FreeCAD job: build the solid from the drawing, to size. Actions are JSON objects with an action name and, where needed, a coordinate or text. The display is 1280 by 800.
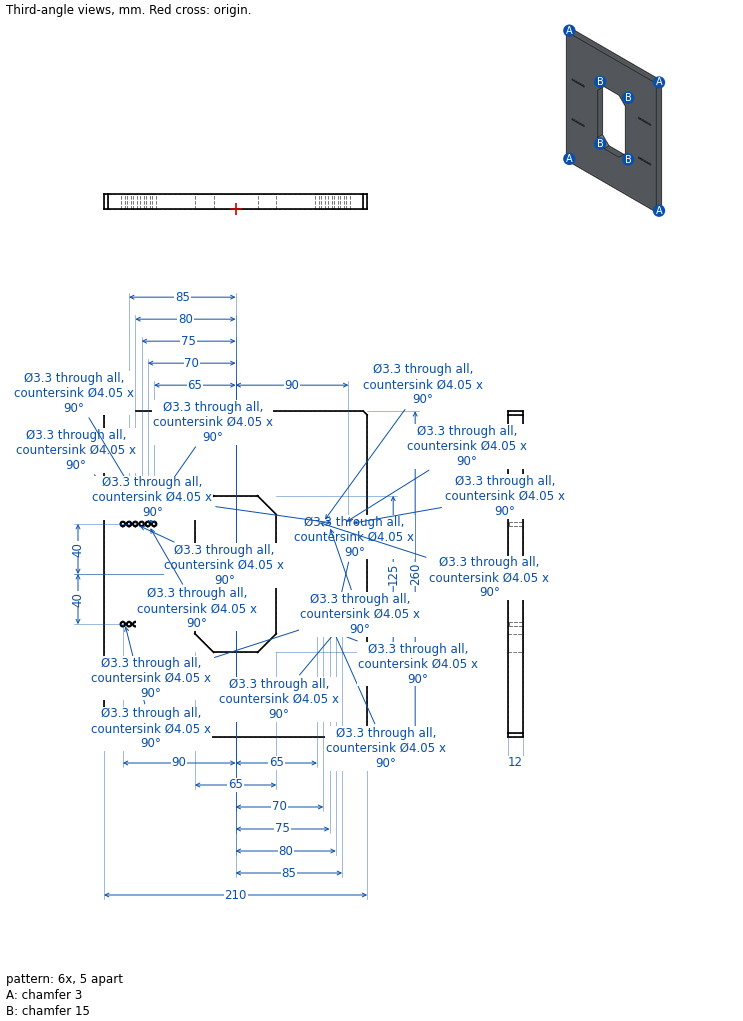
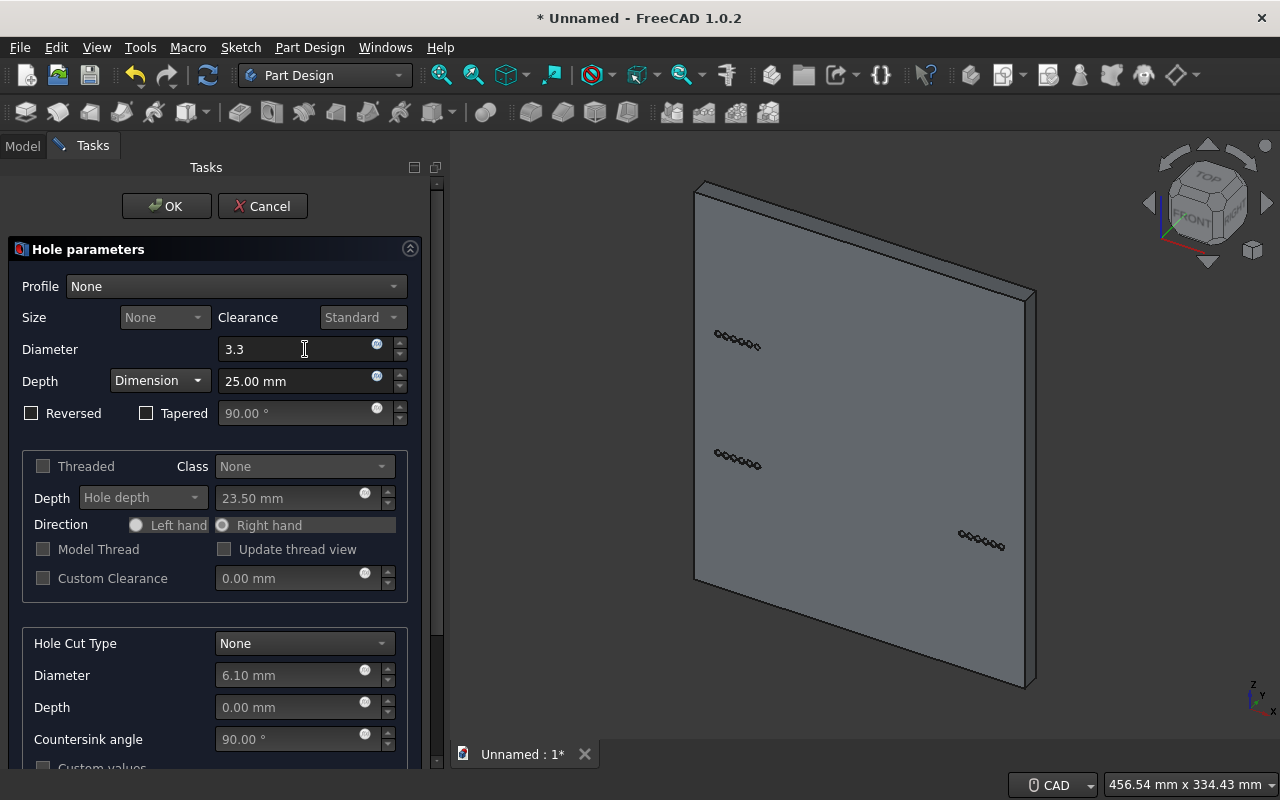
{"action": "left_click", "coordinate": [161, 380]}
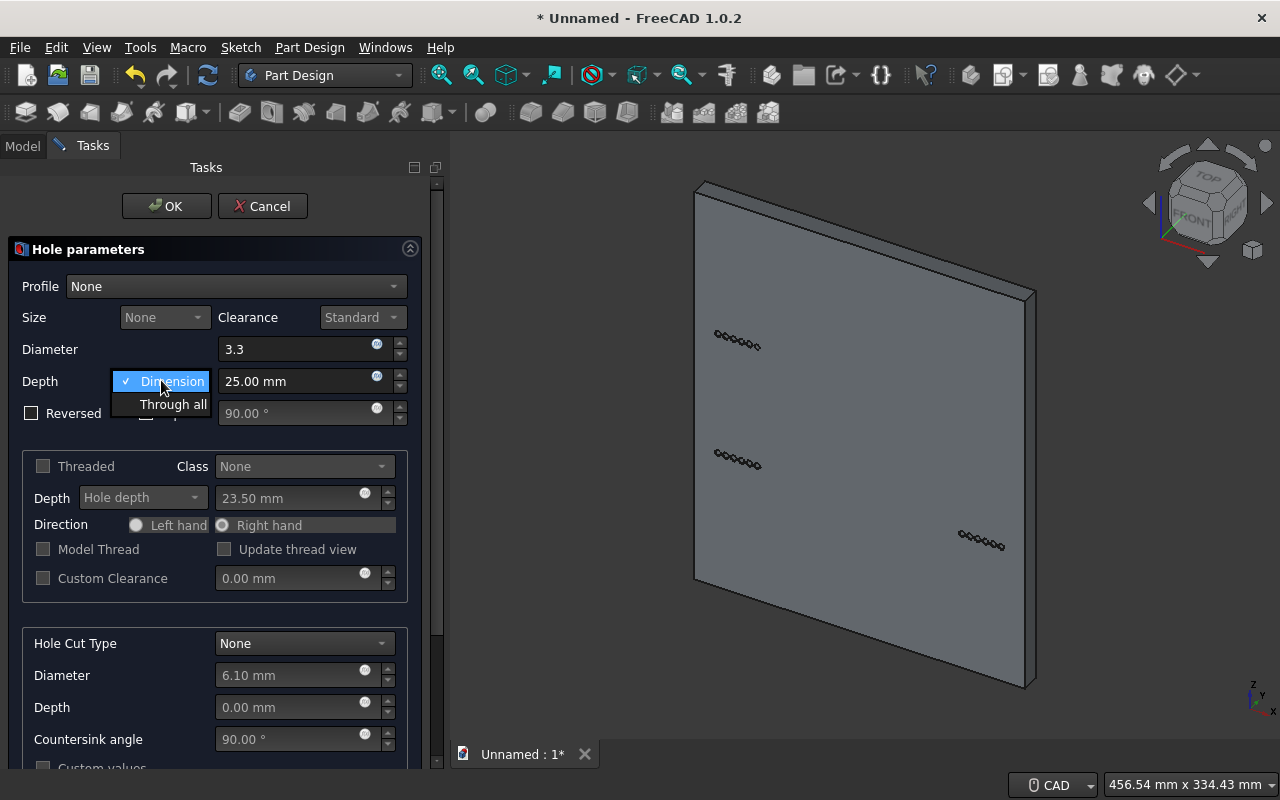
{"action": "left_click", "coordinate": [160, 404]}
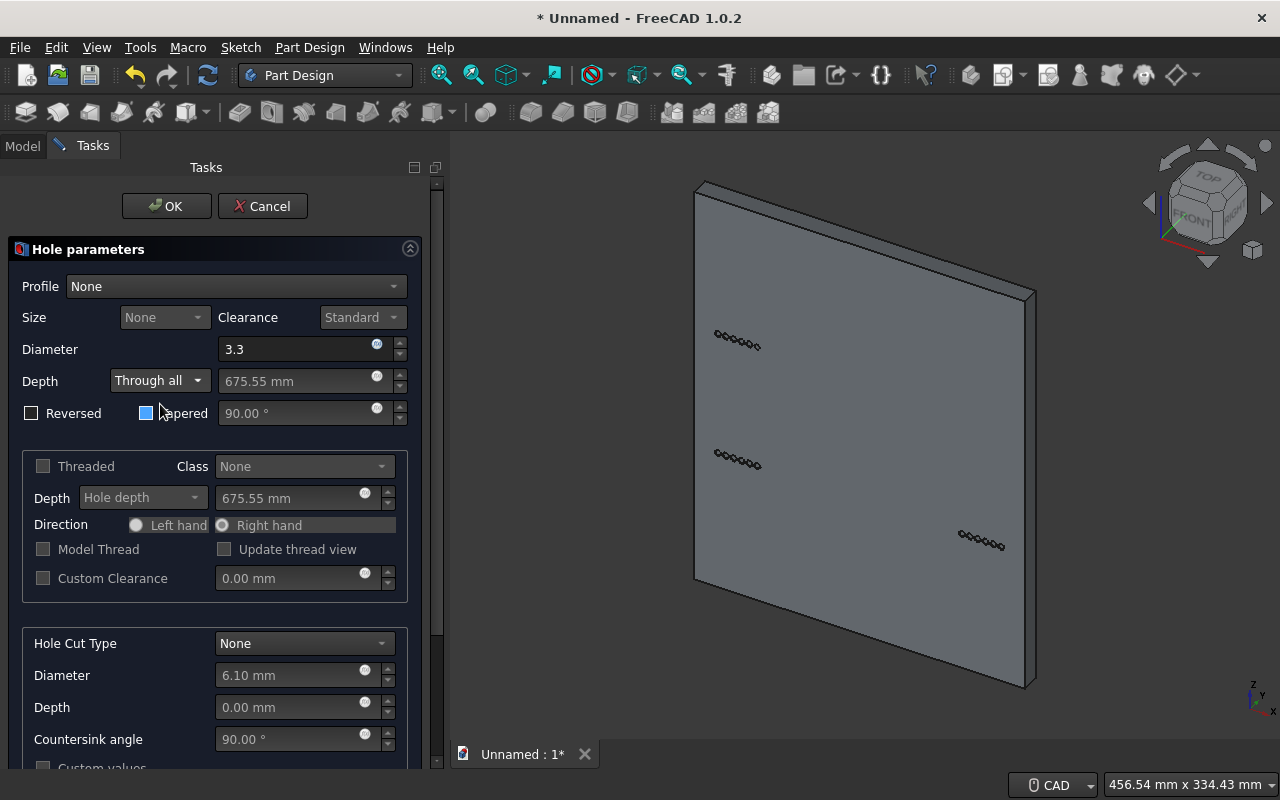
{"action": "left_click", "coordinate": [306, 644]}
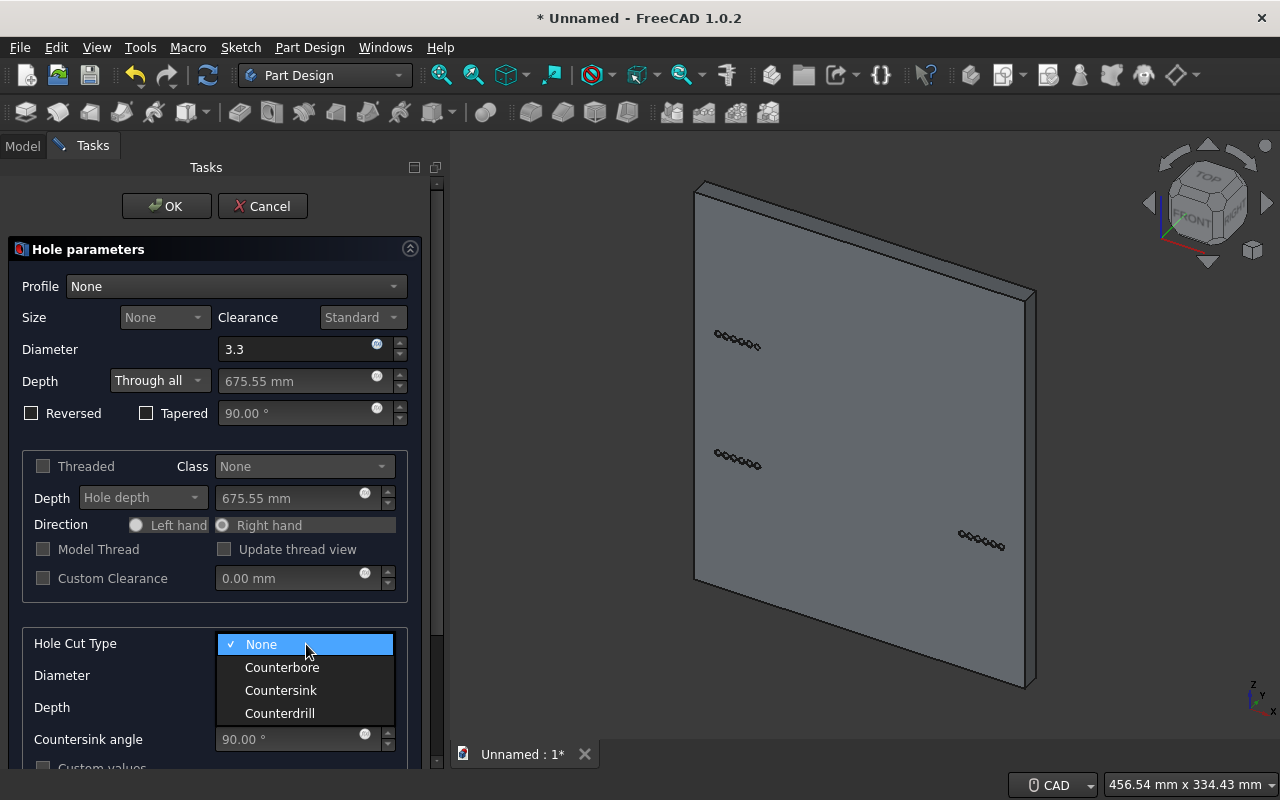
{"action": "left_click", "coordinate": [304, 690]}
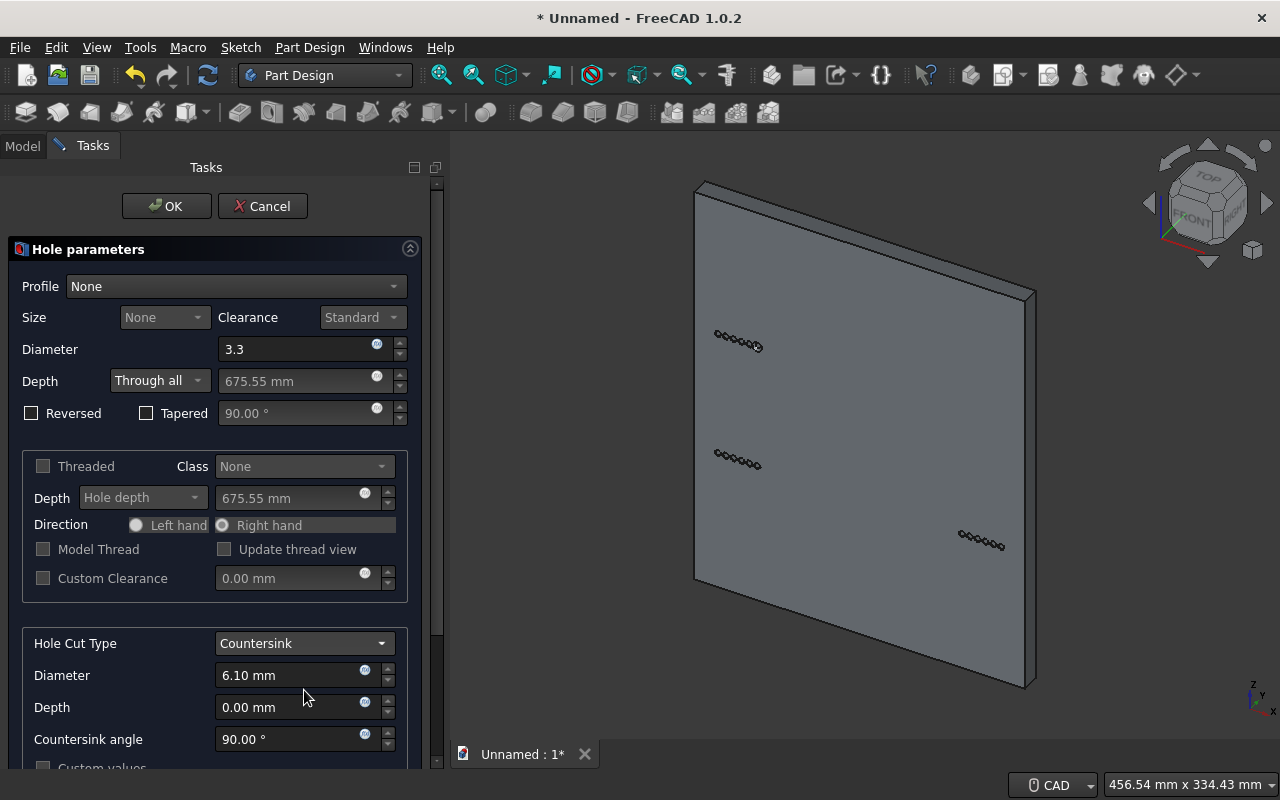
{"action": "triple_click", "coordinate": [298, 675]}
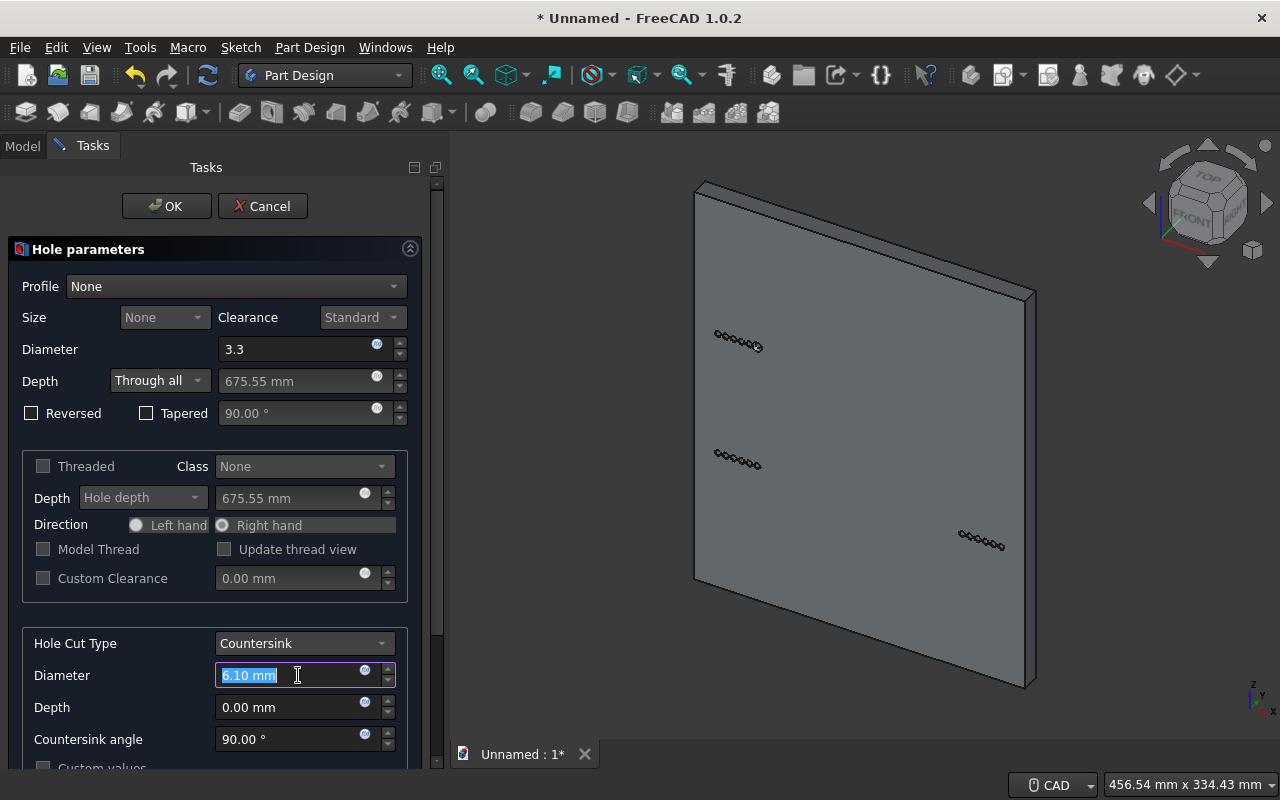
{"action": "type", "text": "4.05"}
{"action": "key", "text": "Tab"}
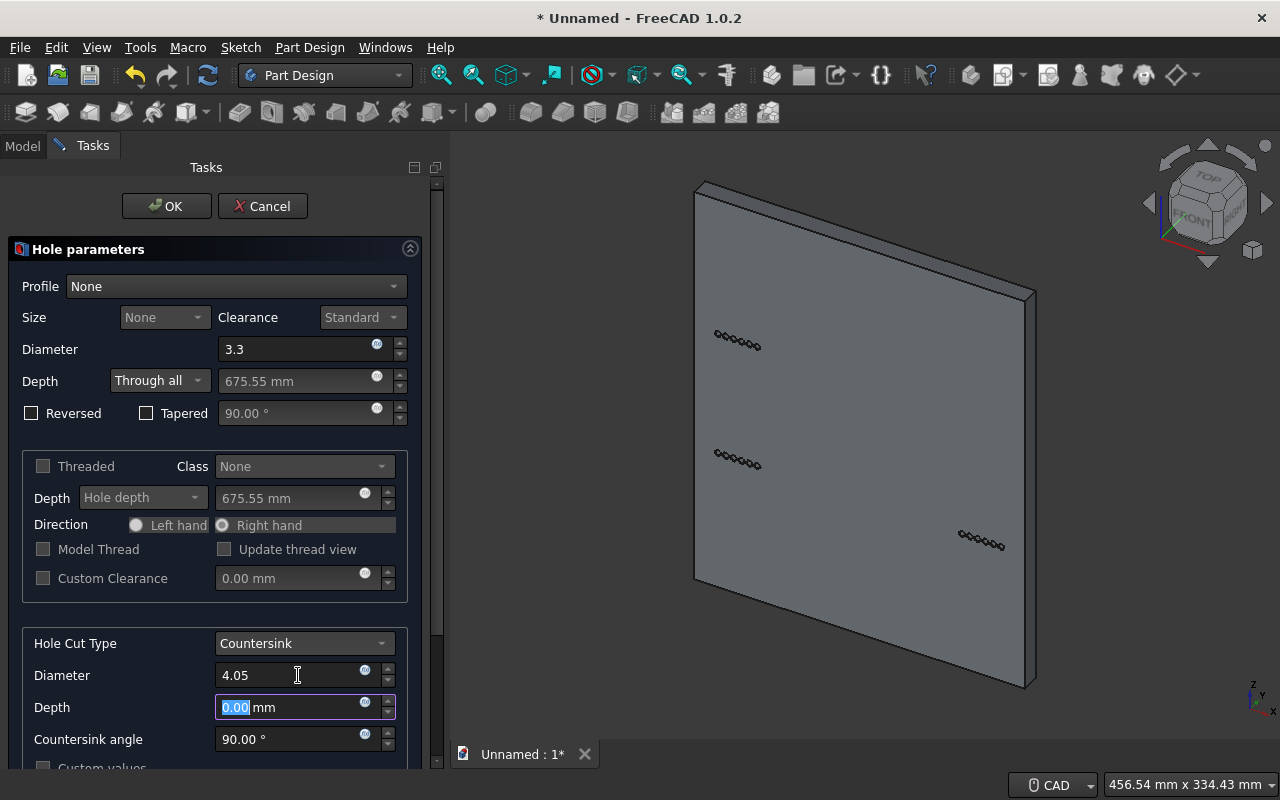
{"action": "left_click", "coordinate": [167, 206]}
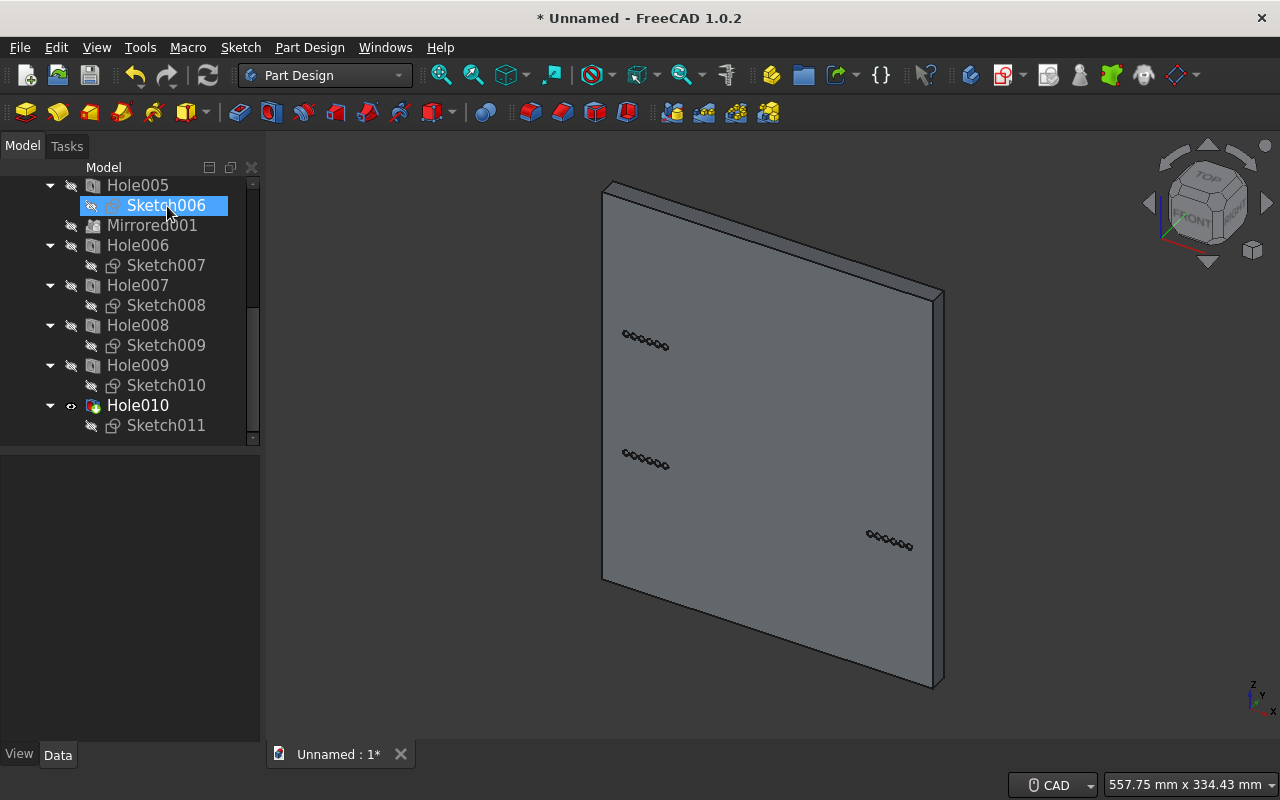
{"action": "left_click", "coordinate": [815, 400]}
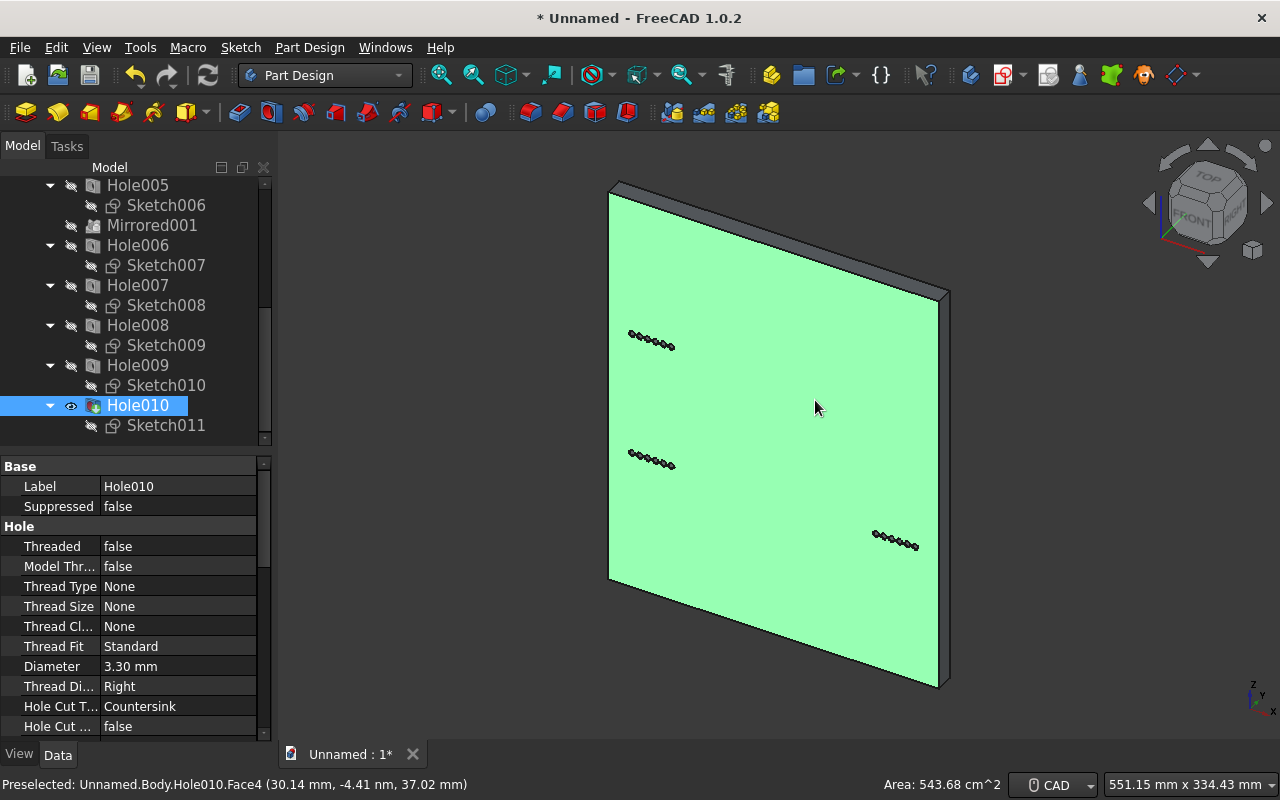
{"action": "left_click", "coordinate": [1004, 76]}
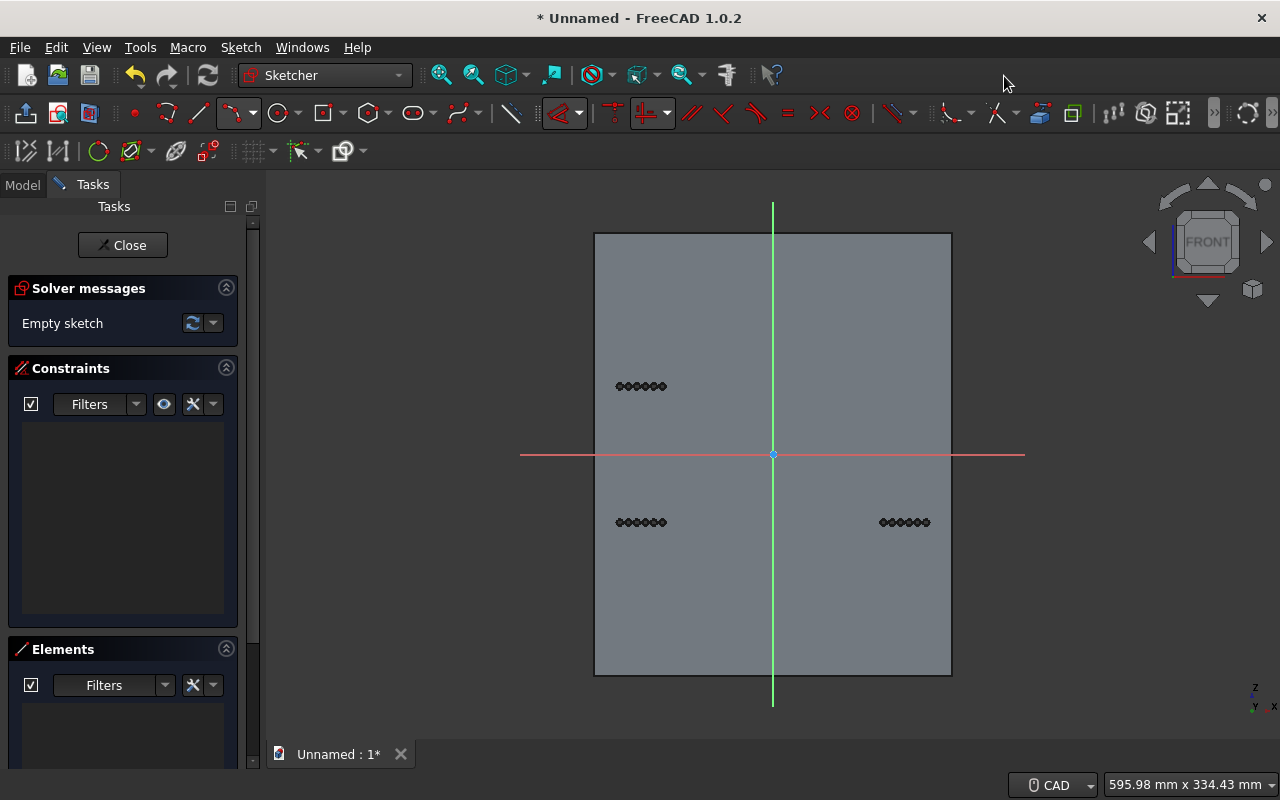
{"action": "scroll", "coordinate": [938, 383], "scroll_direction": "up", "scroll_amount": 15}